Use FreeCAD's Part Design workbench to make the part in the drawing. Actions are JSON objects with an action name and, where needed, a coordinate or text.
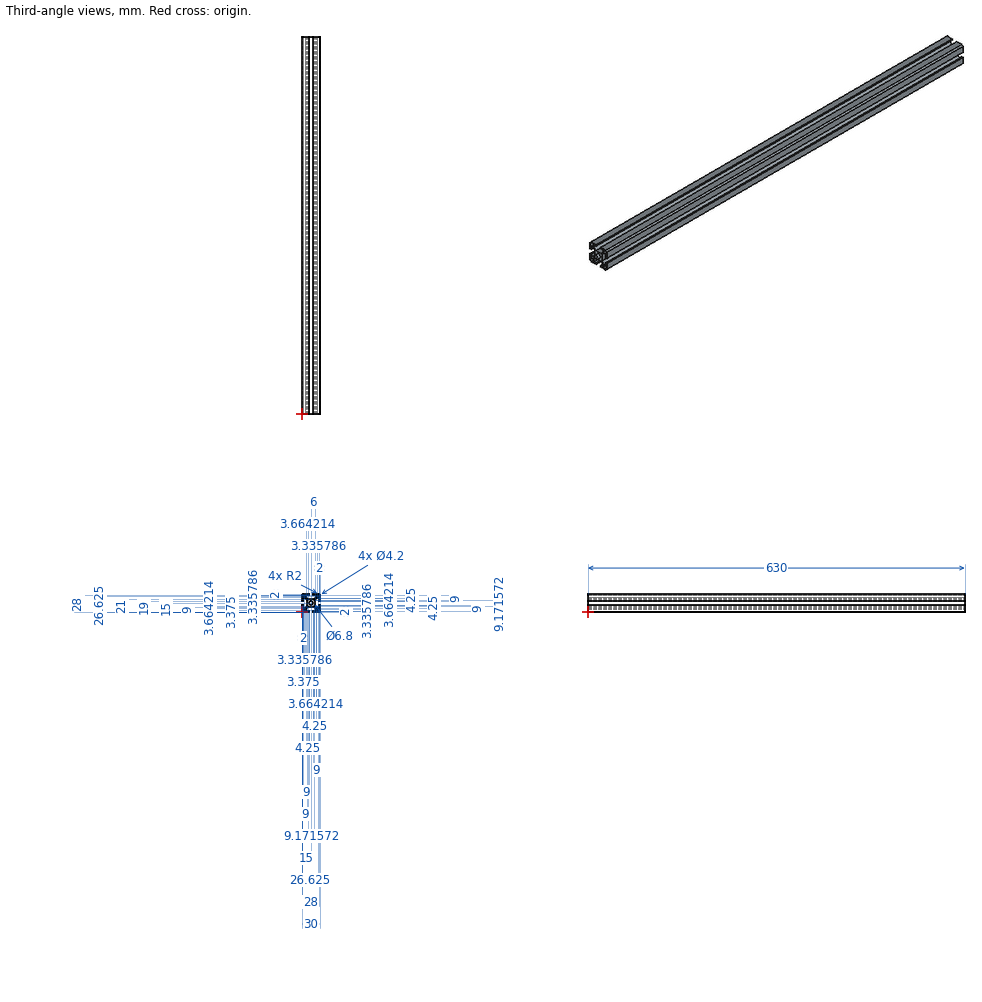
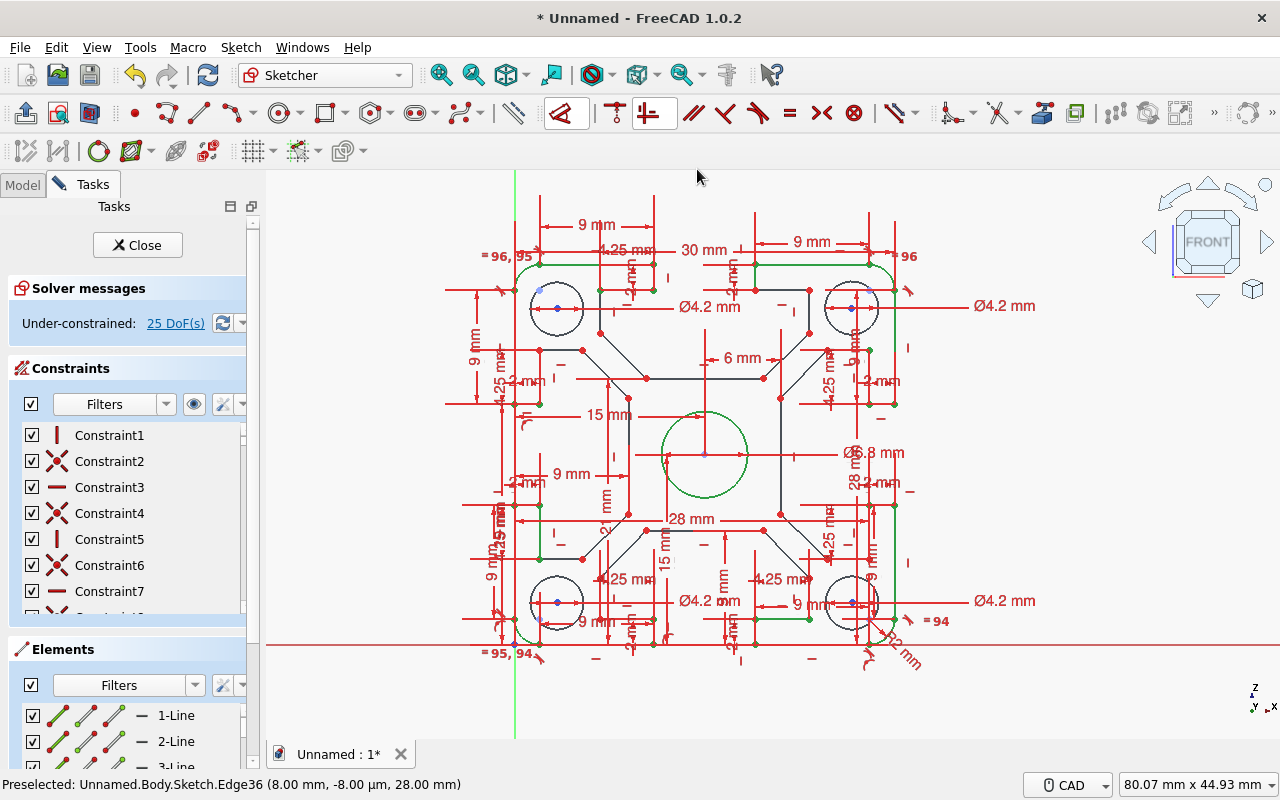
{"action": "left_click", "coordinate": [793, 290]}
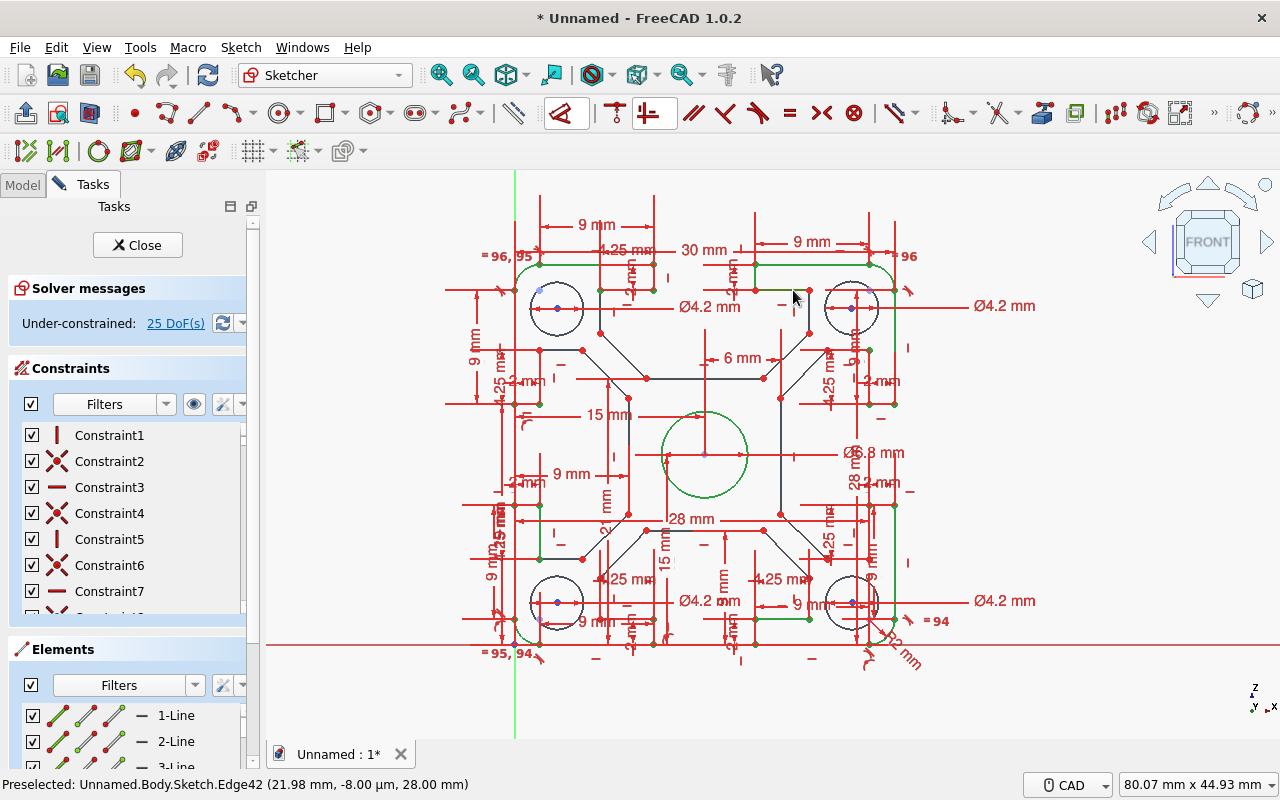
{"action": "key", "text": "l"}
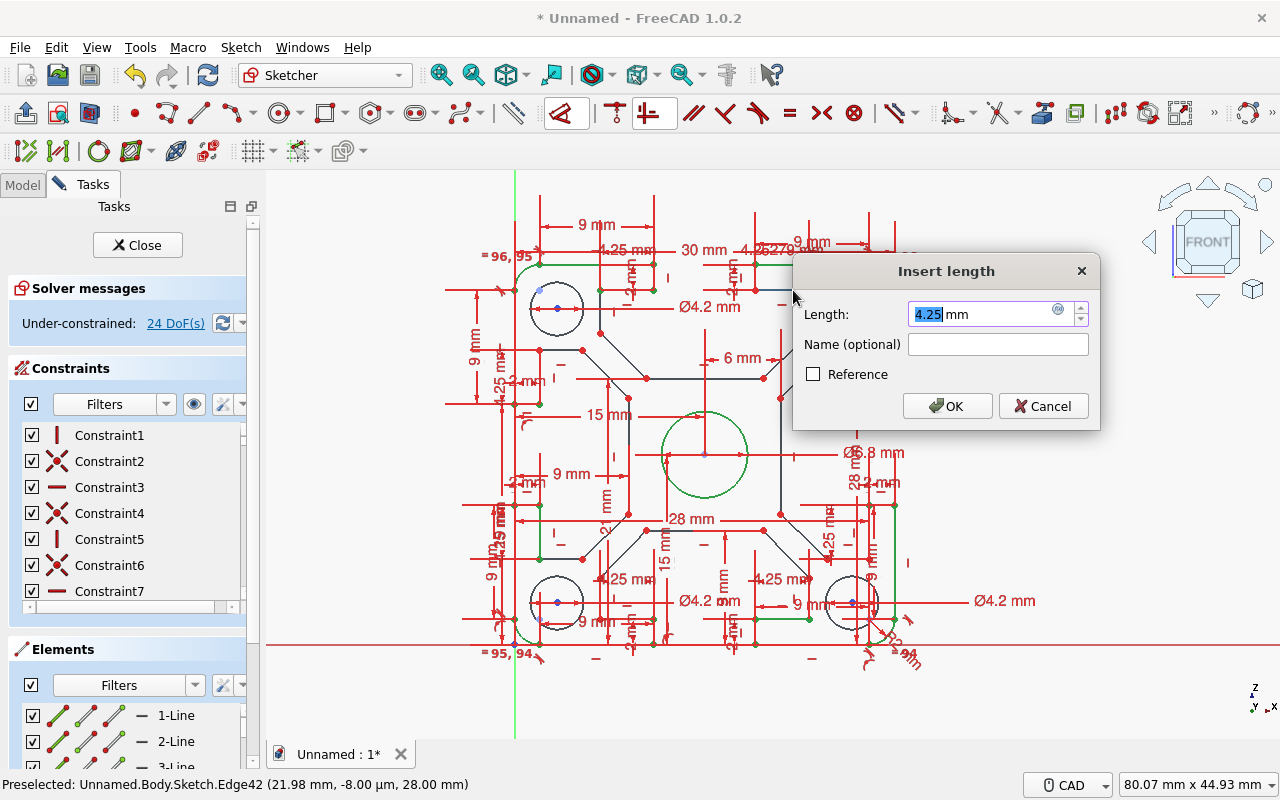
{"action": "type", "text": "4.25"}
{"action": "key", "text": "Return"}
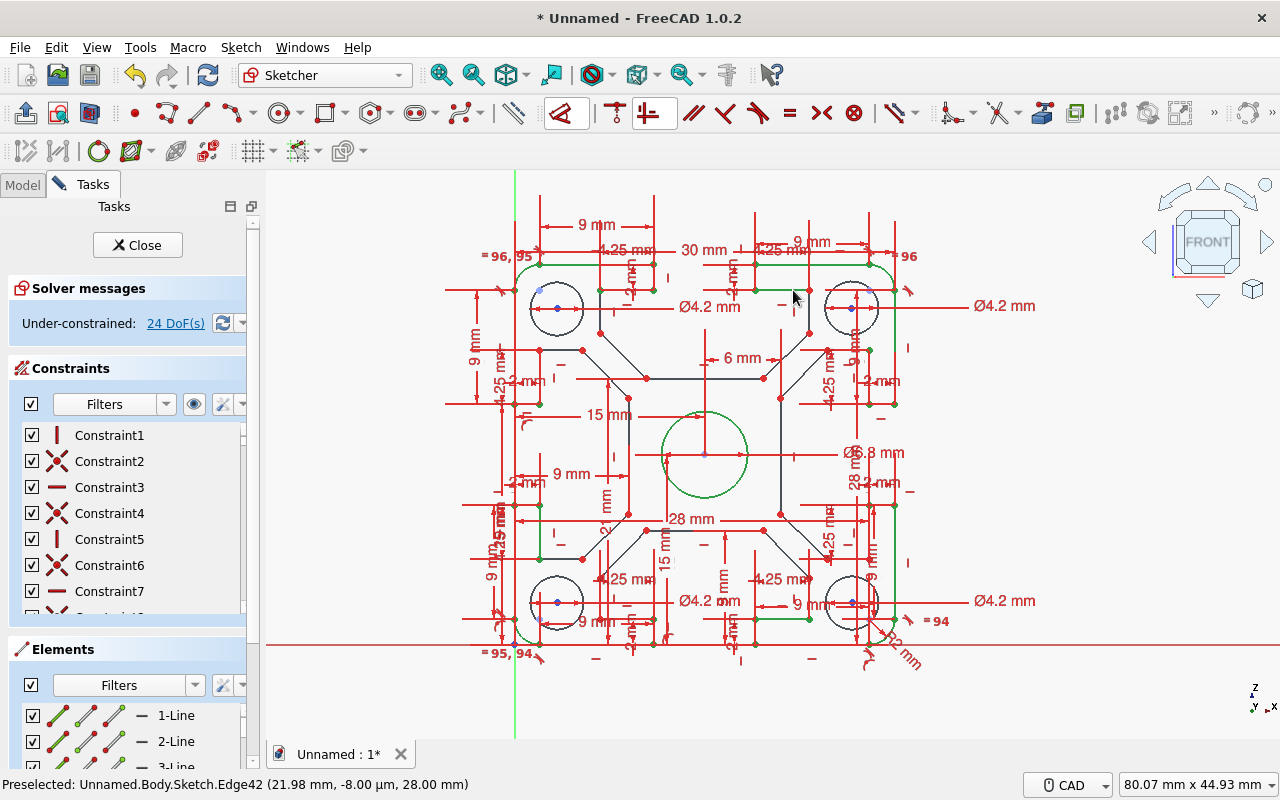
{"action": "left_click", "coordinate": [557, 309]}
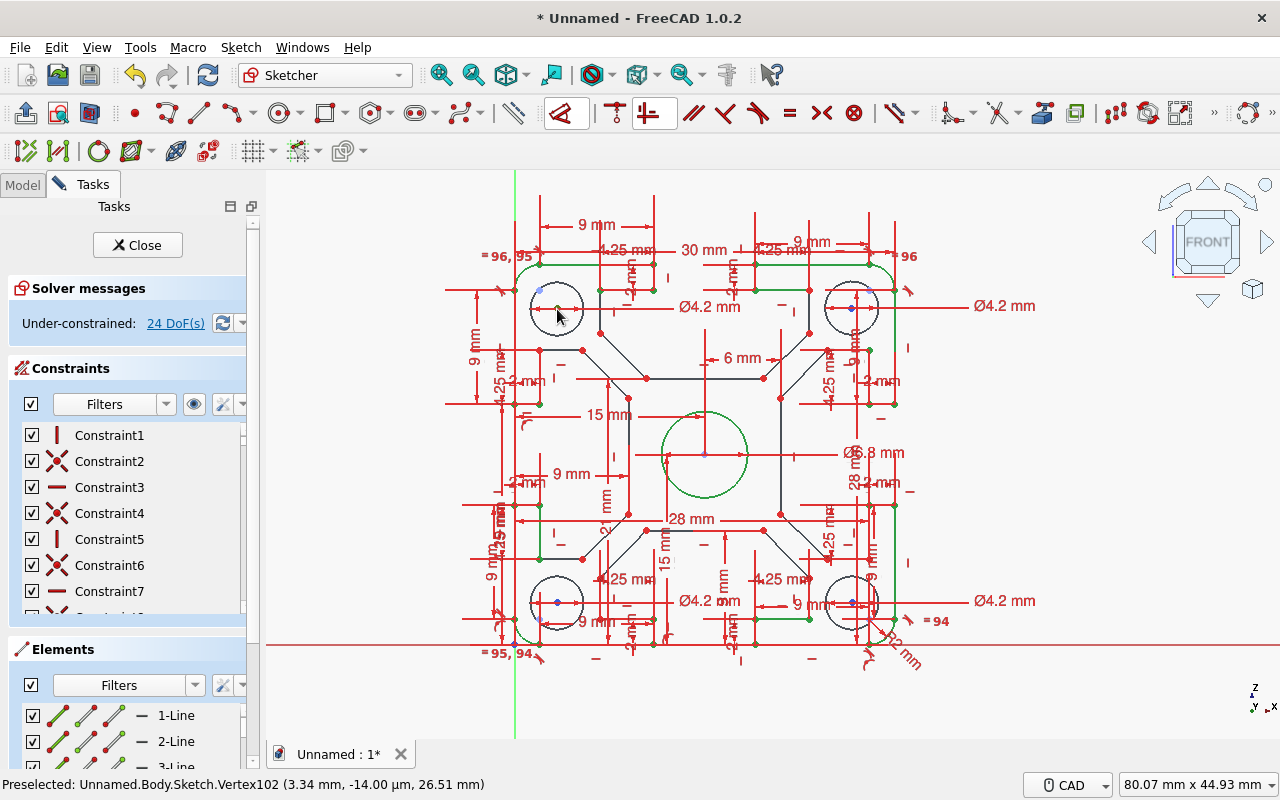
{"action": "key", "text": "l"}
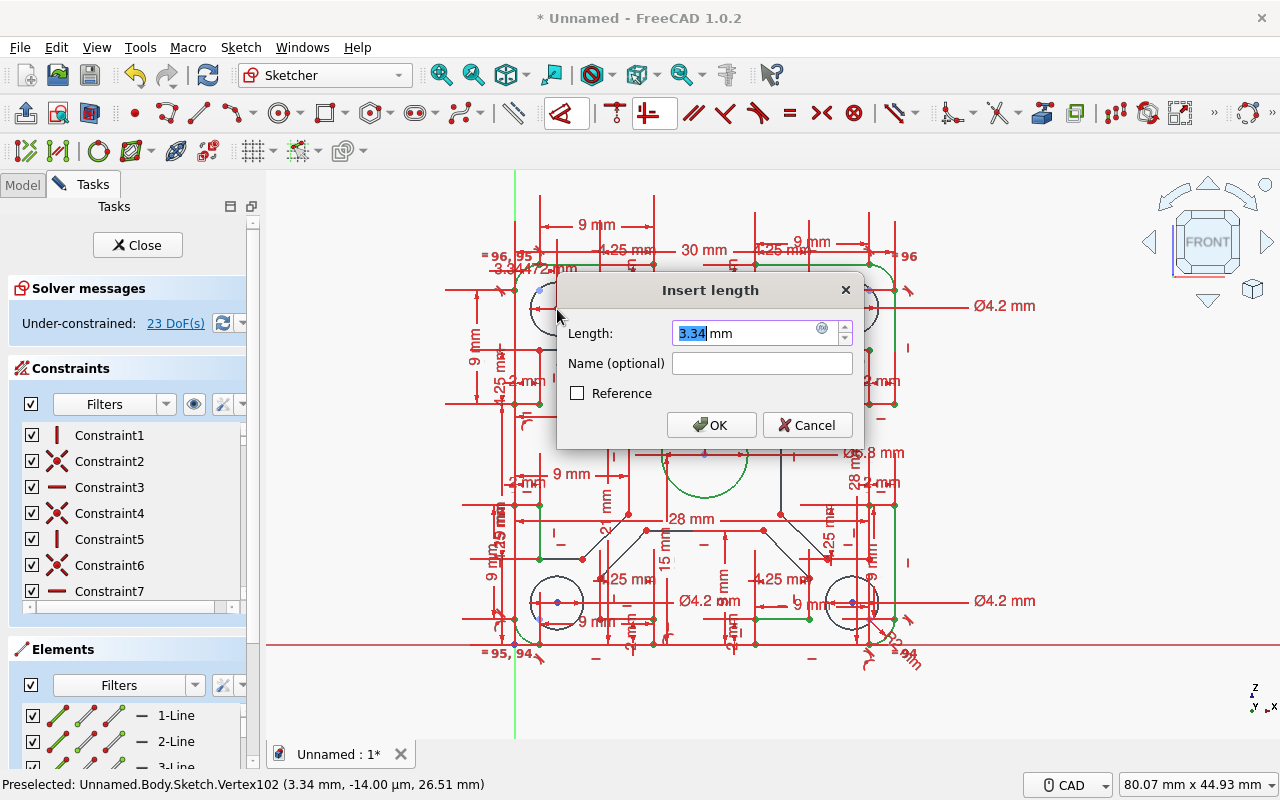
{"action": "type", "text": "3.375"}
{"action": "key", "text": "Return"}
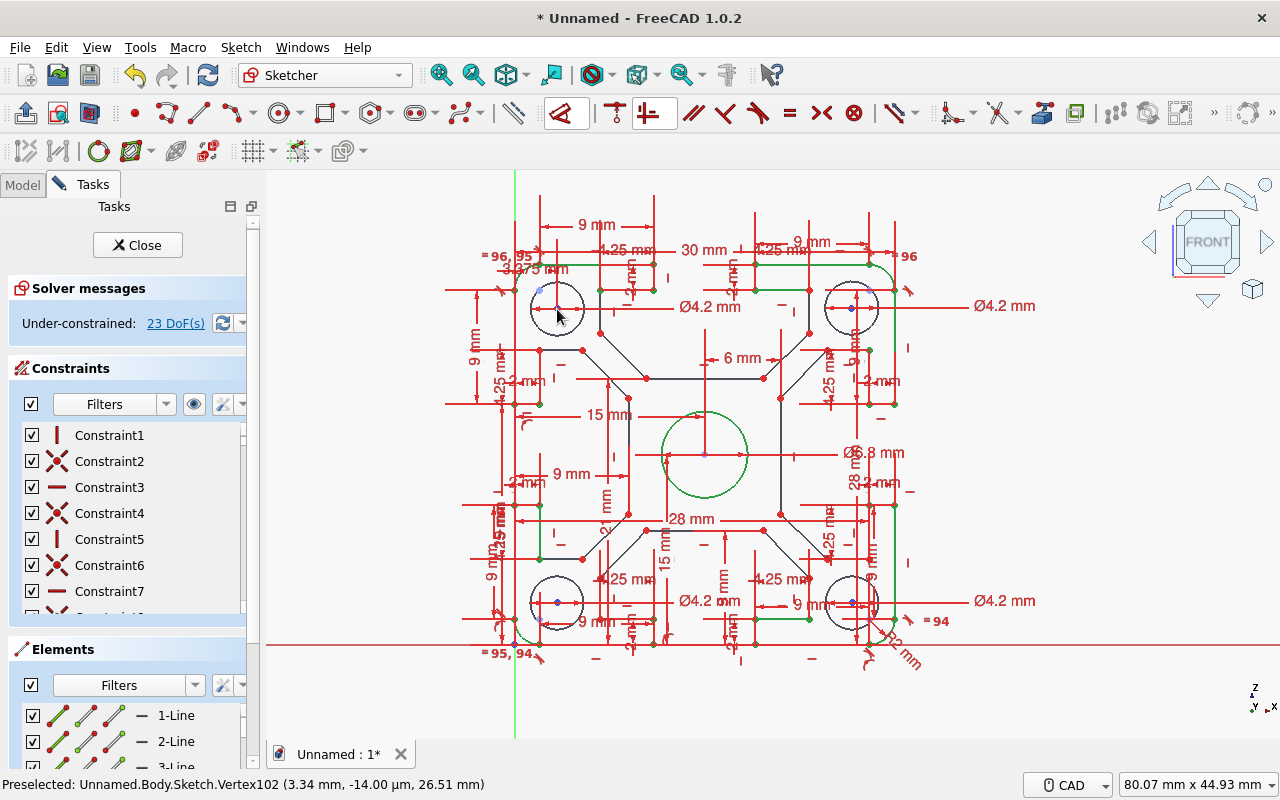
{"action": "left_click", "coordinate": [852, 603]}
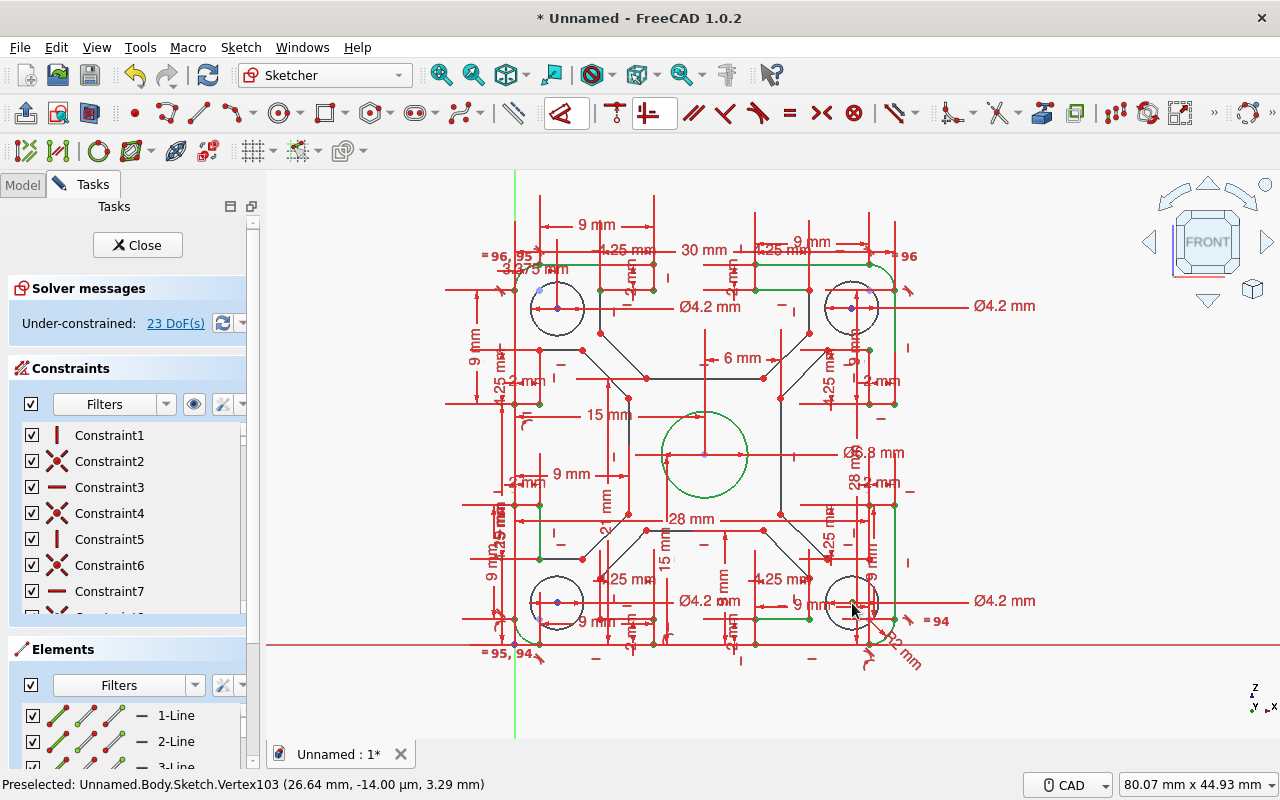
{"action": "key", "text": "i"}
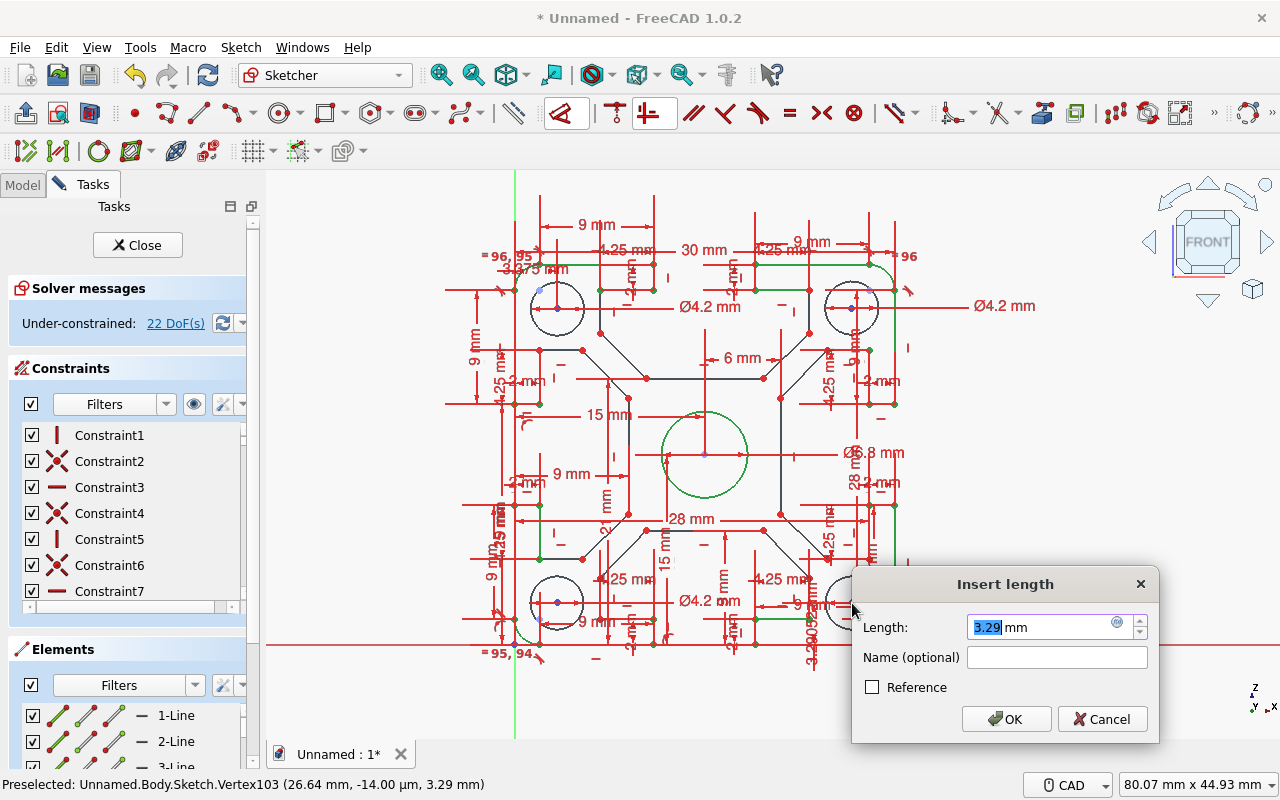
{"action": "type", "text": "3.375"}
{"action": "key", "text": "Return"}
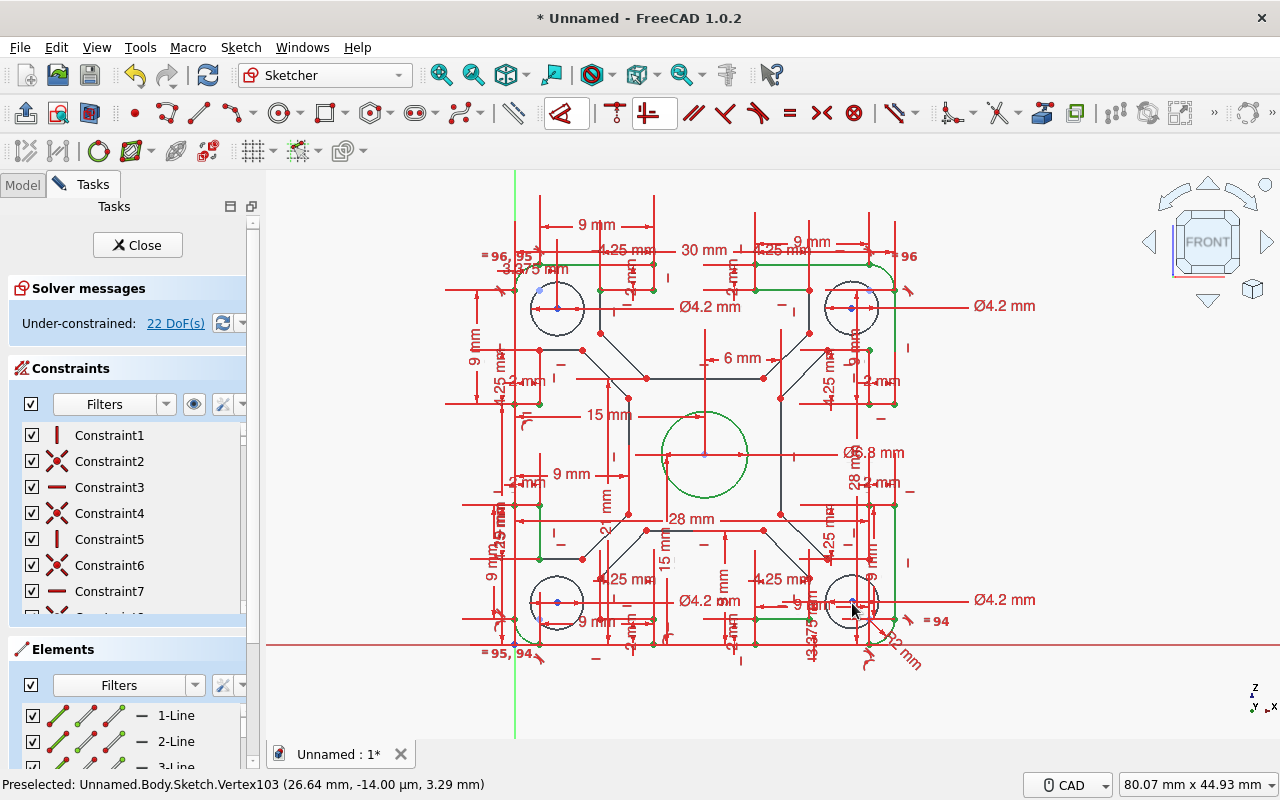
{"action": "left_click", "coordinate": [557, 603]}